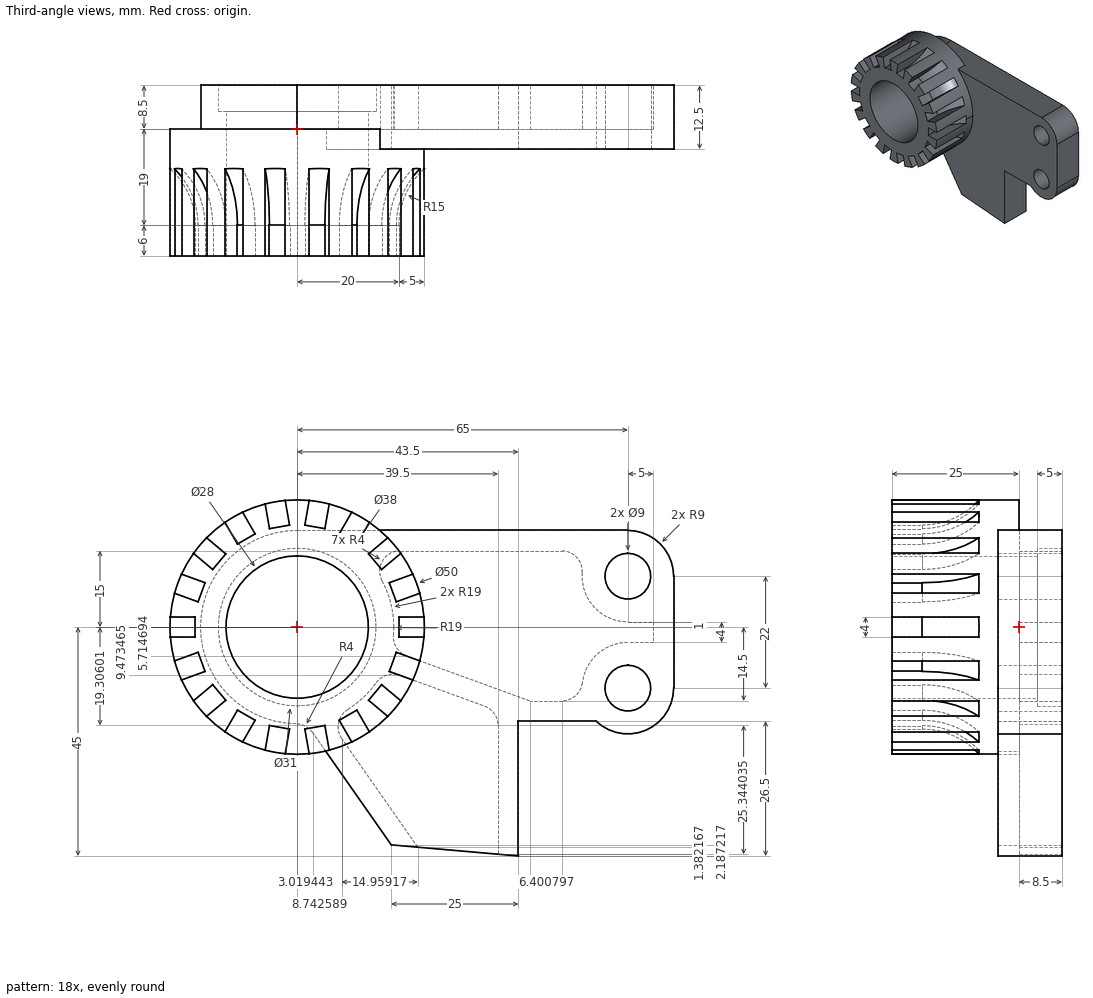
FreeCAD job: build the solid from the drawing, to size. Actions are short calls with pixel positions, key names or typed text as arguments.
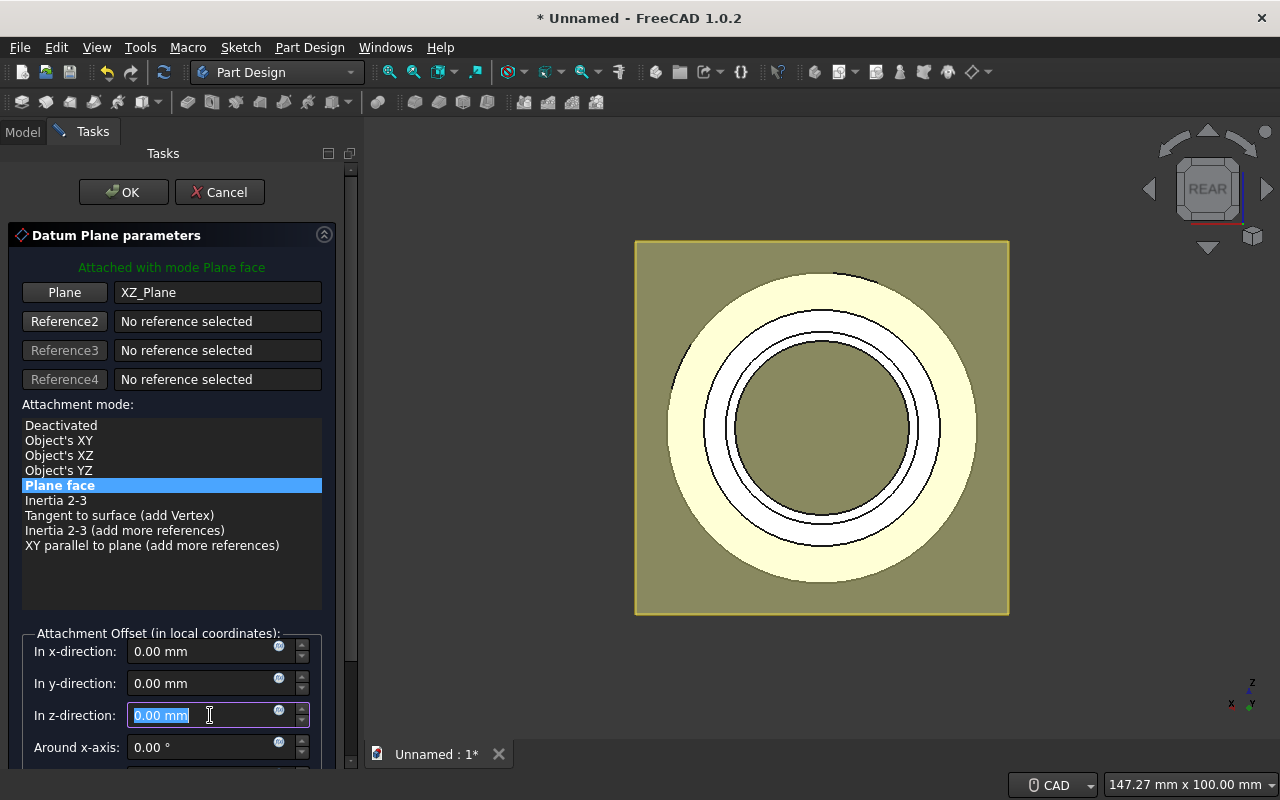
text(4)
key(Tab)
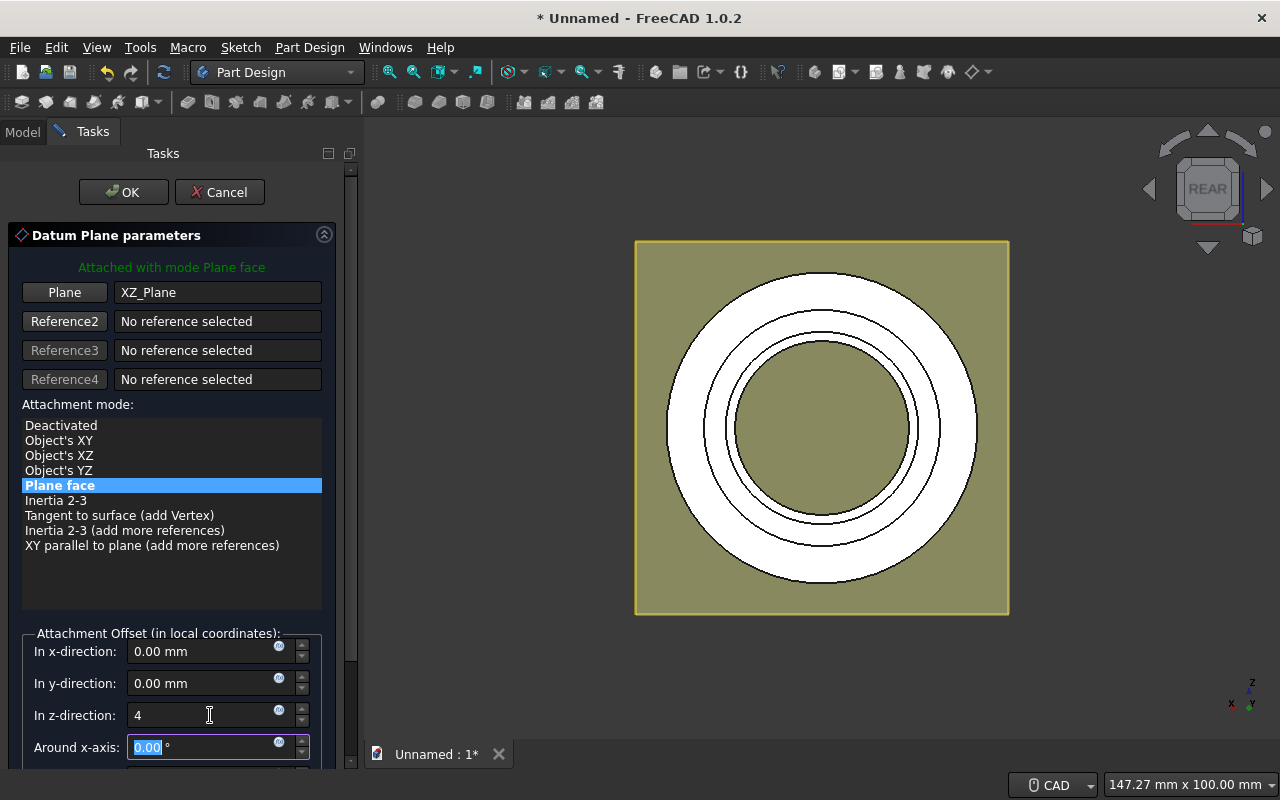
click(124, 192)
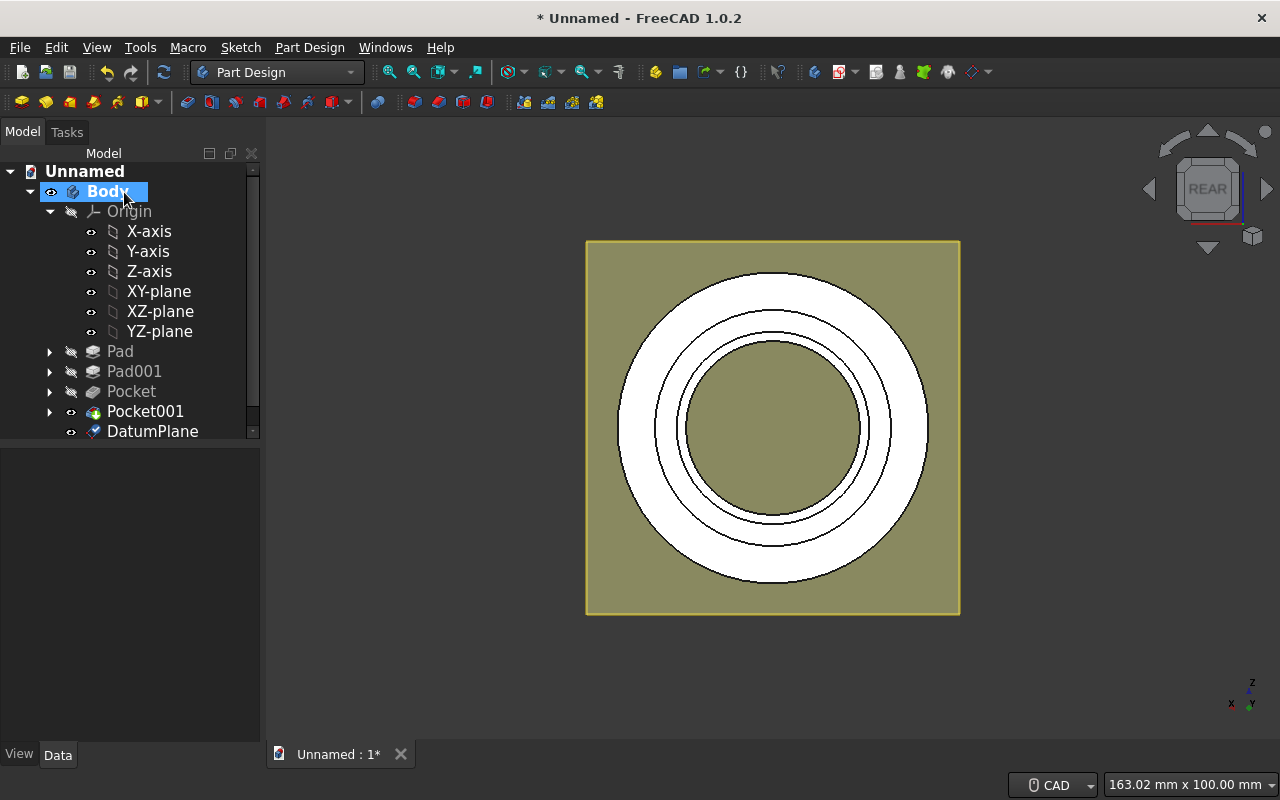
click(116, 432)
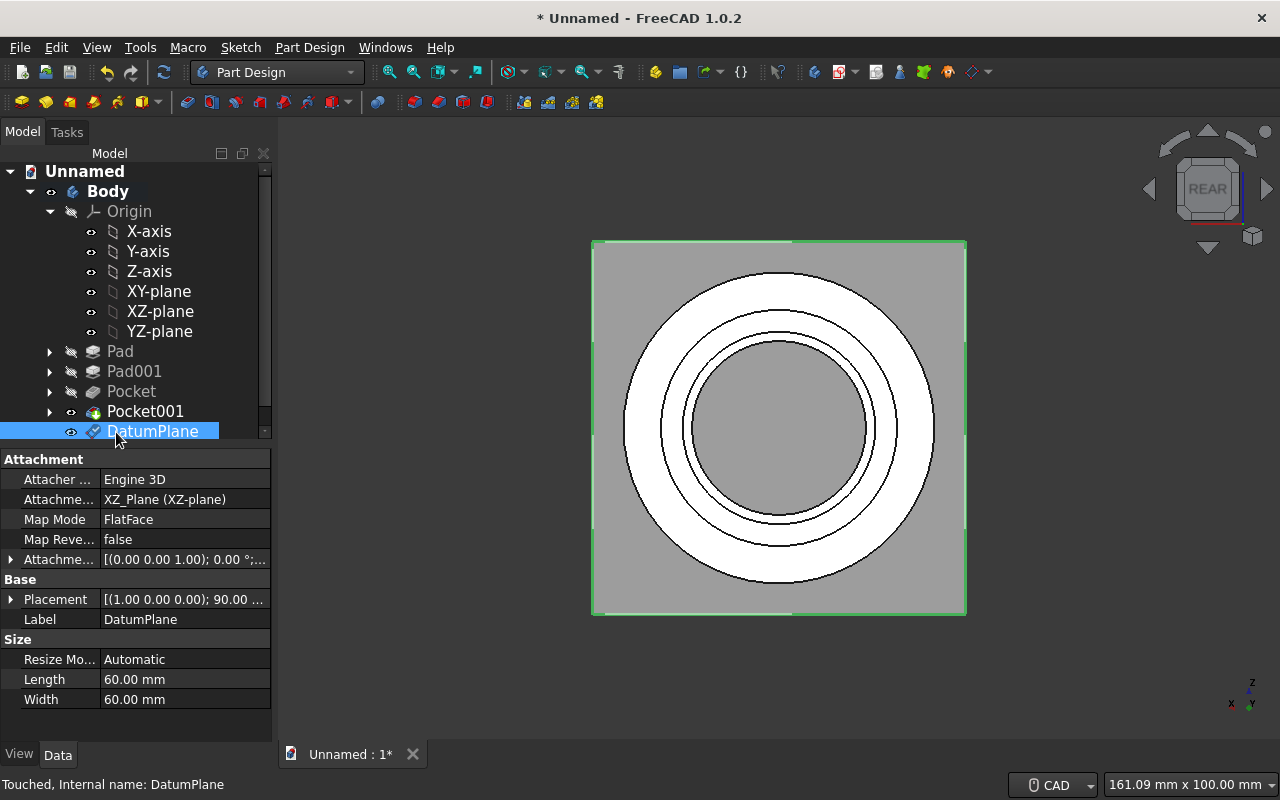
click(840, 72)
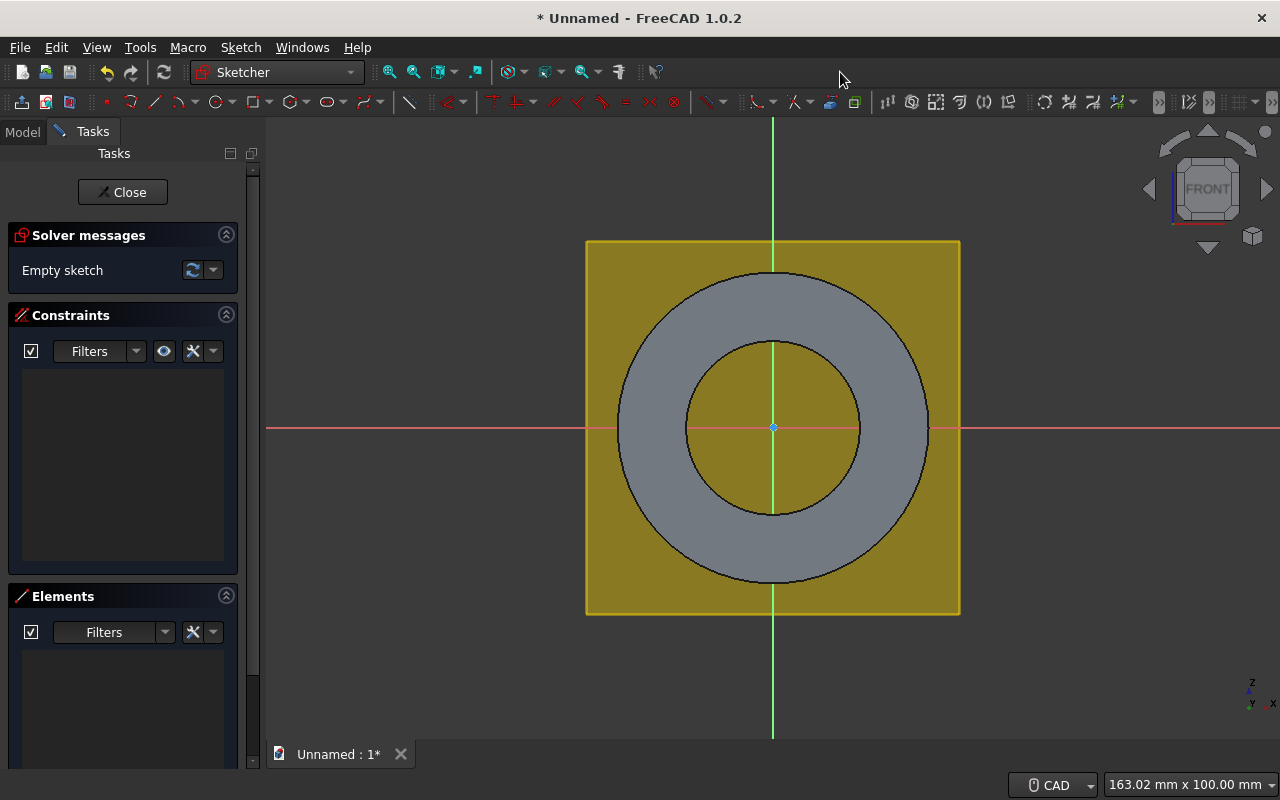
click(70, 102)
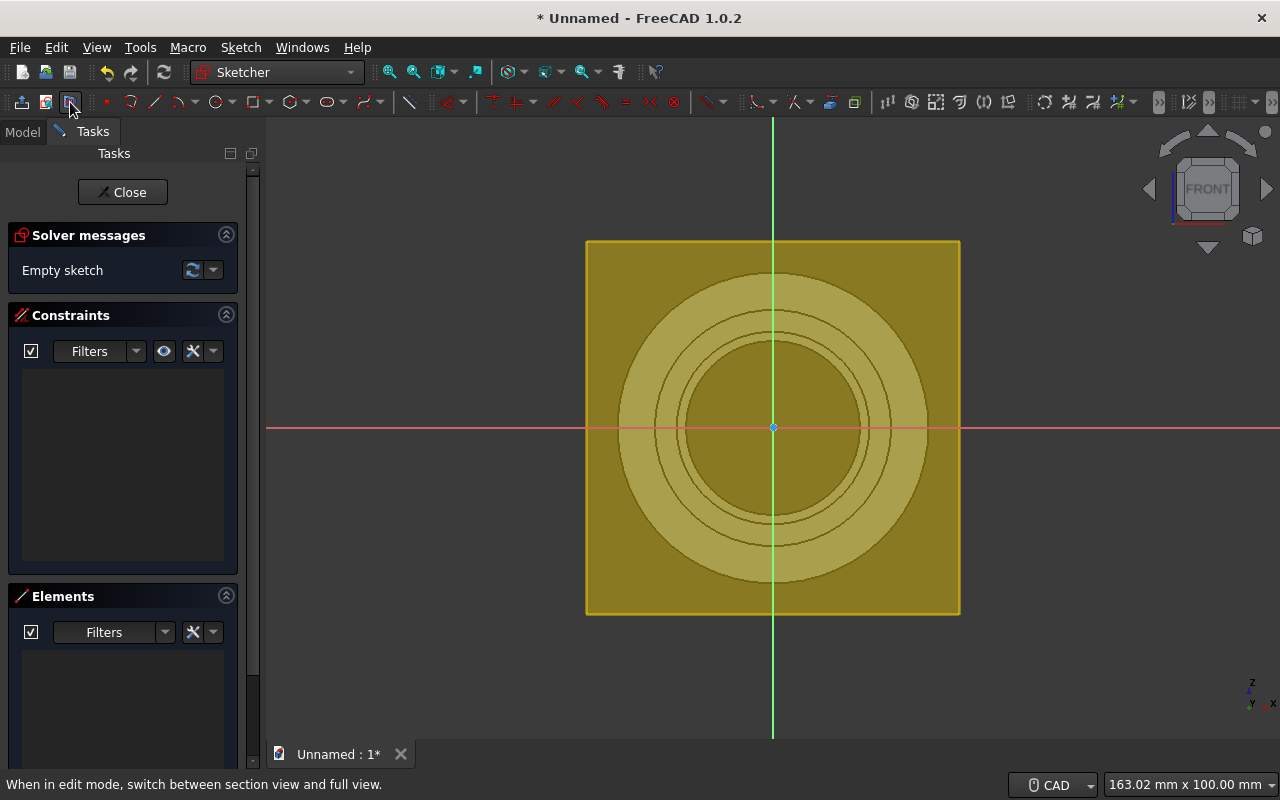
scroll(294, 145, down, 1)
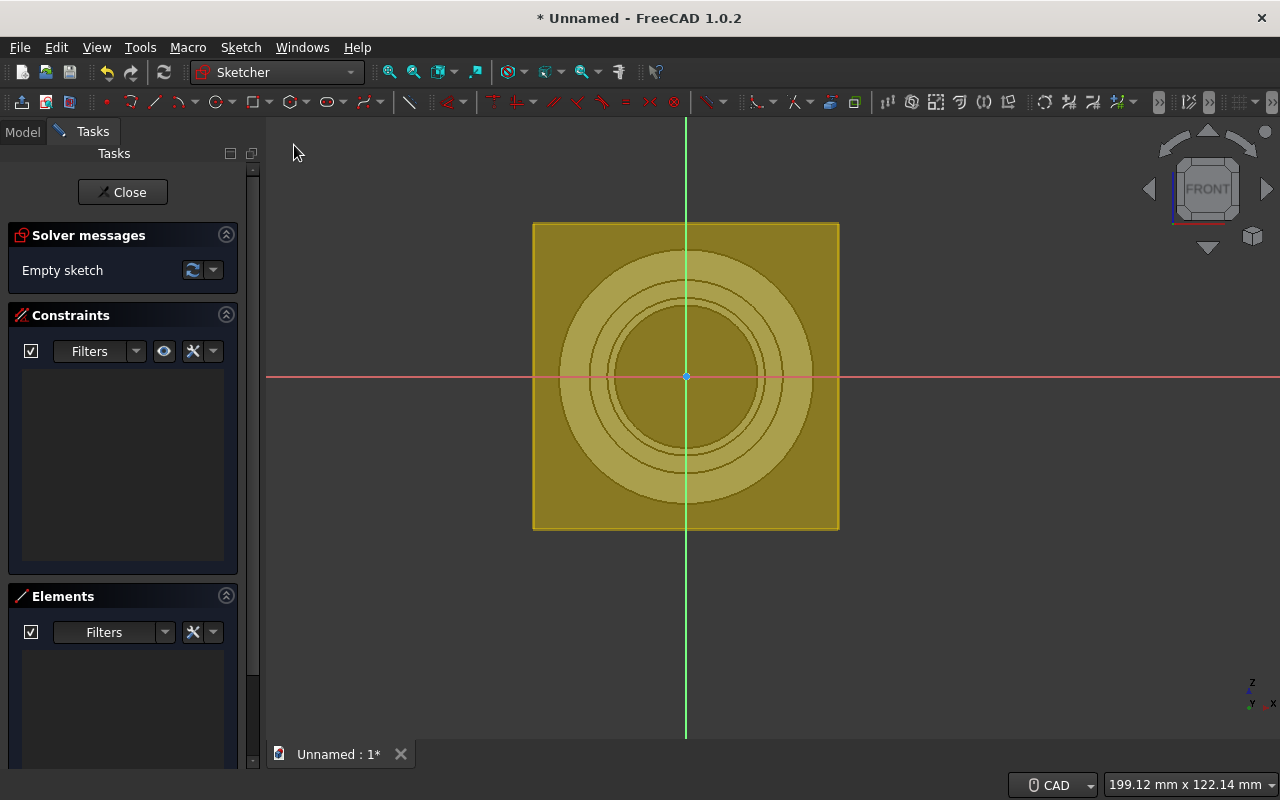
click(156, 102)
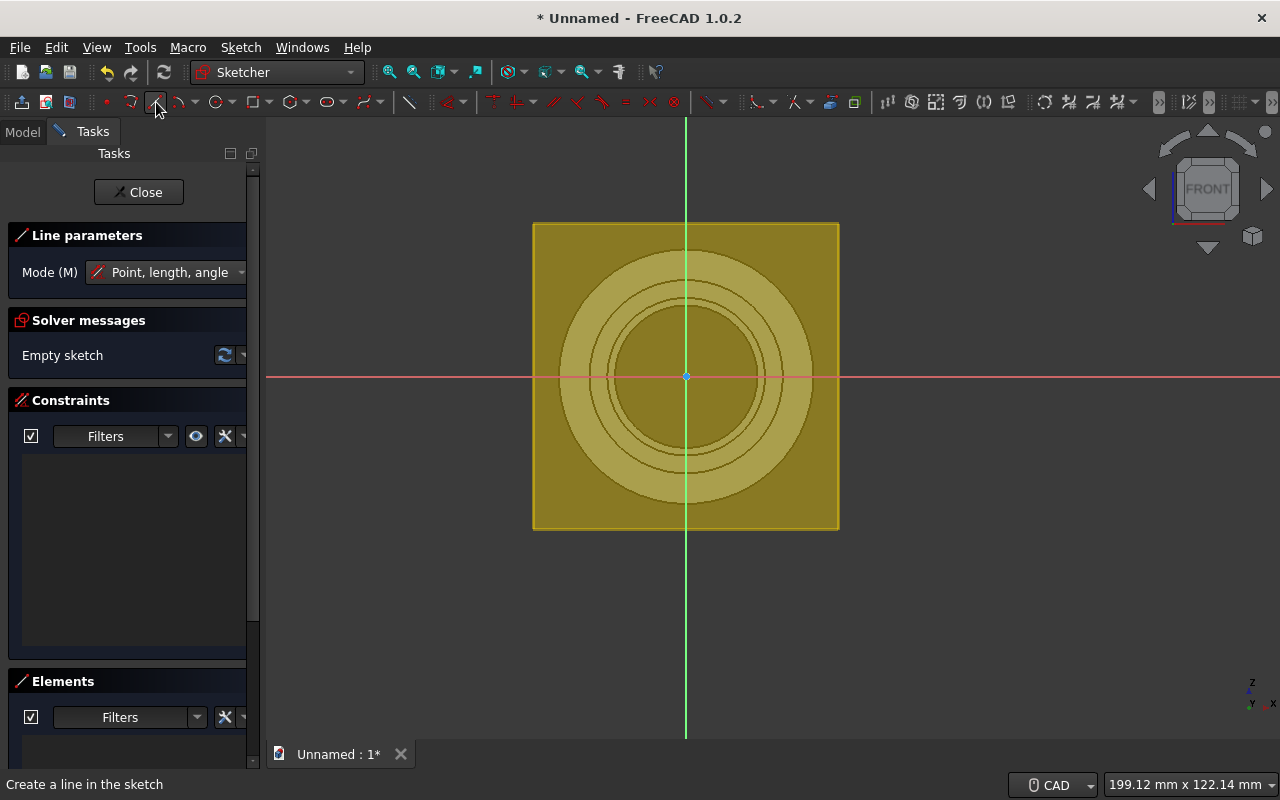
click(686, 280)
click(1017, 280)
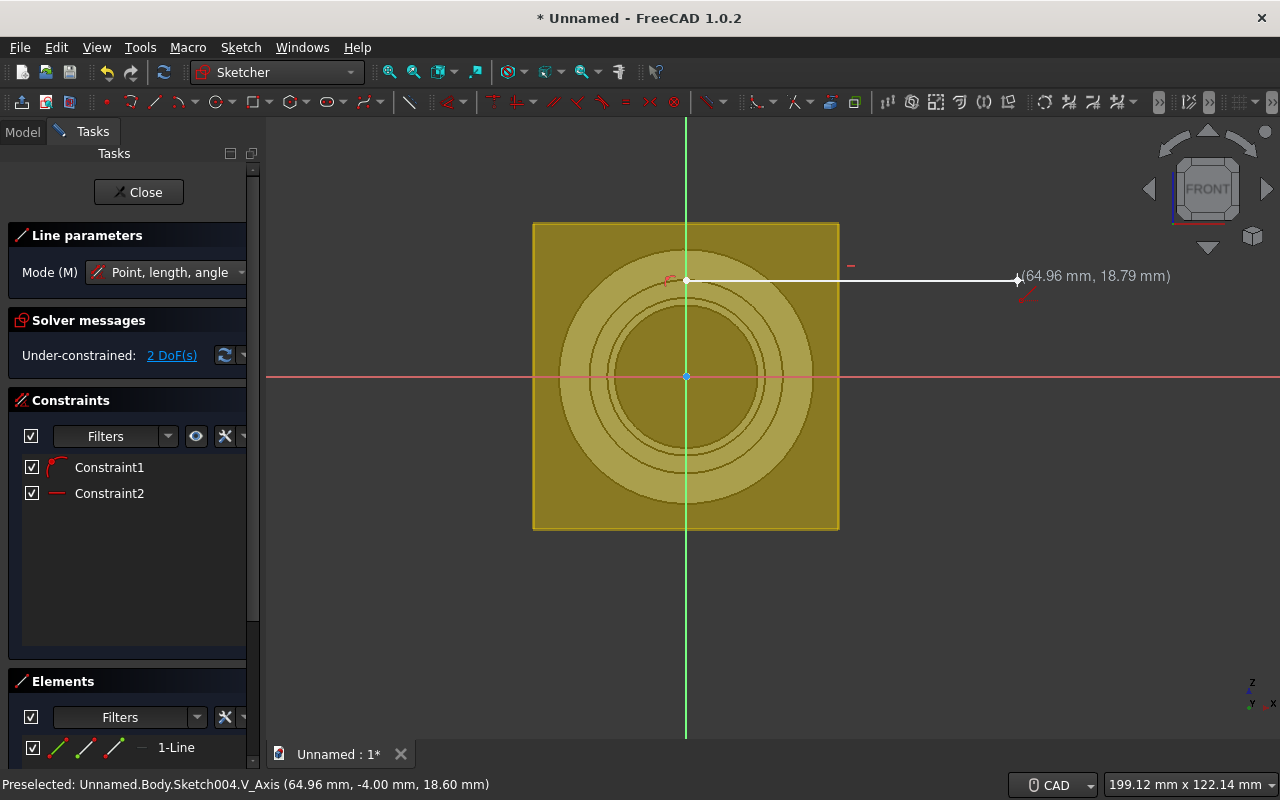
click(1063, 326)
click(1063, 438)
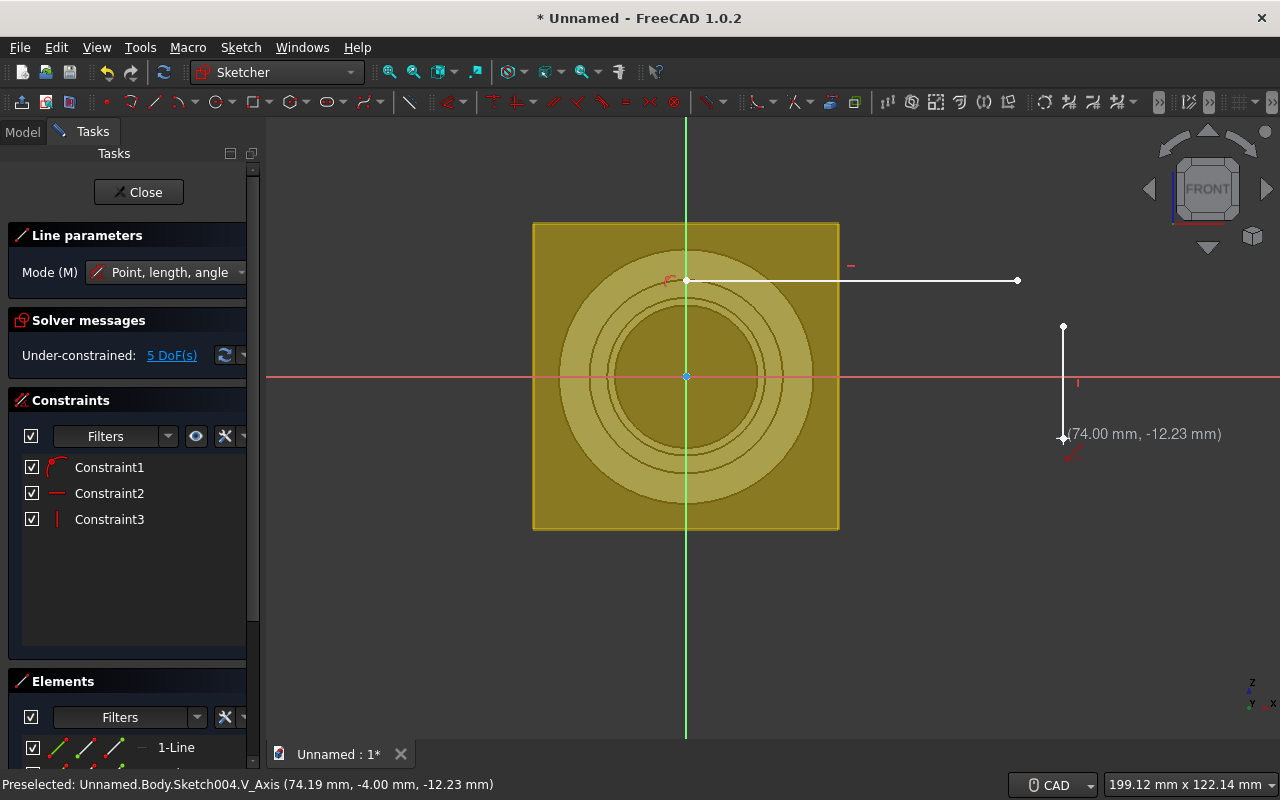
click(132, 102)